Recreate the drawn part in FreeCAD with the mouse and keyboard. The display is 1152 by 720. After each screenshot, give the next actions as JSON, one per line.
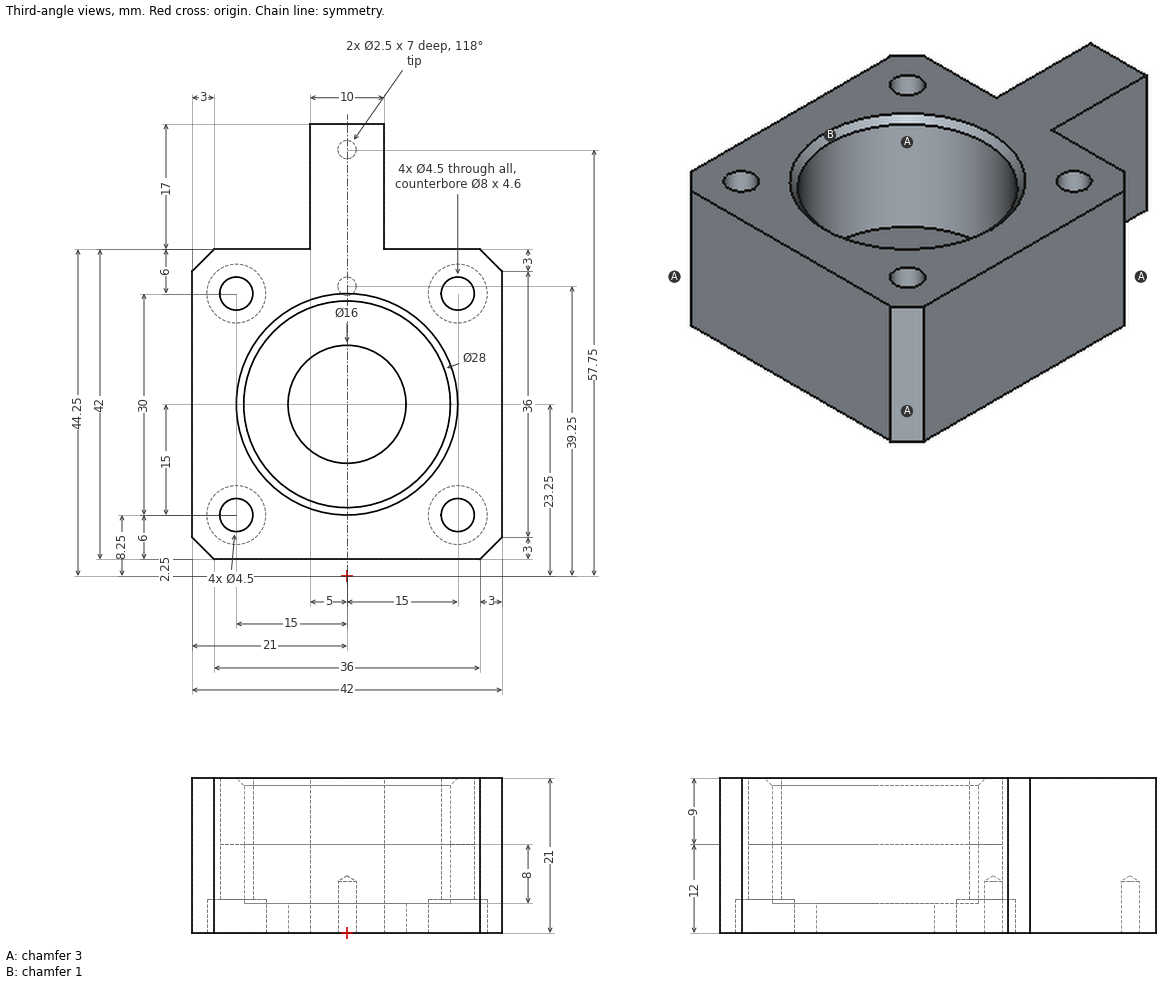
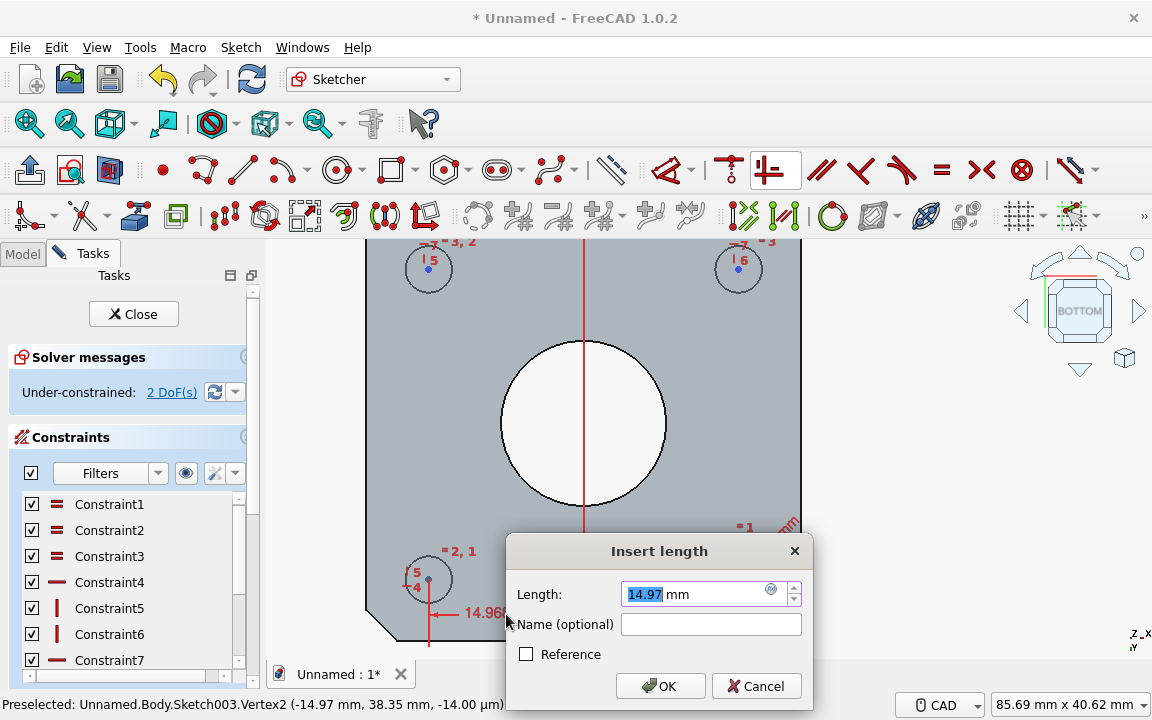
{"action": "type", "text": "15"}
{"action": "key", "text": "Return"}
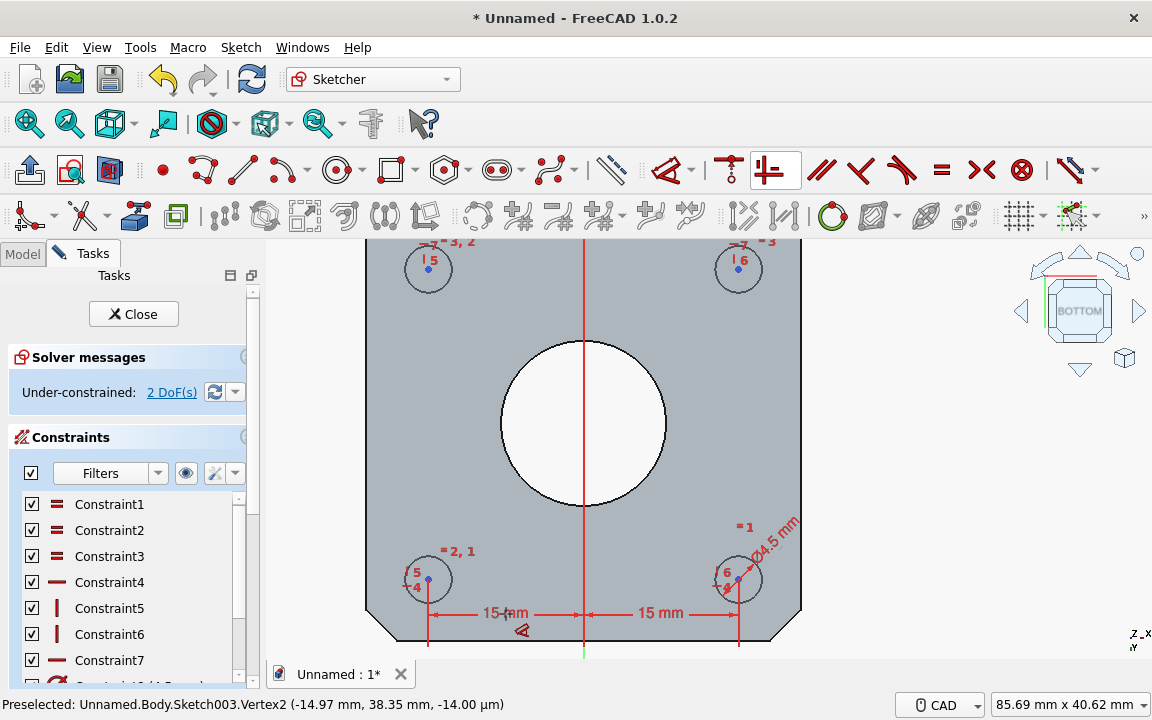
{"action": "left_click", "coordinate": [428, 580]}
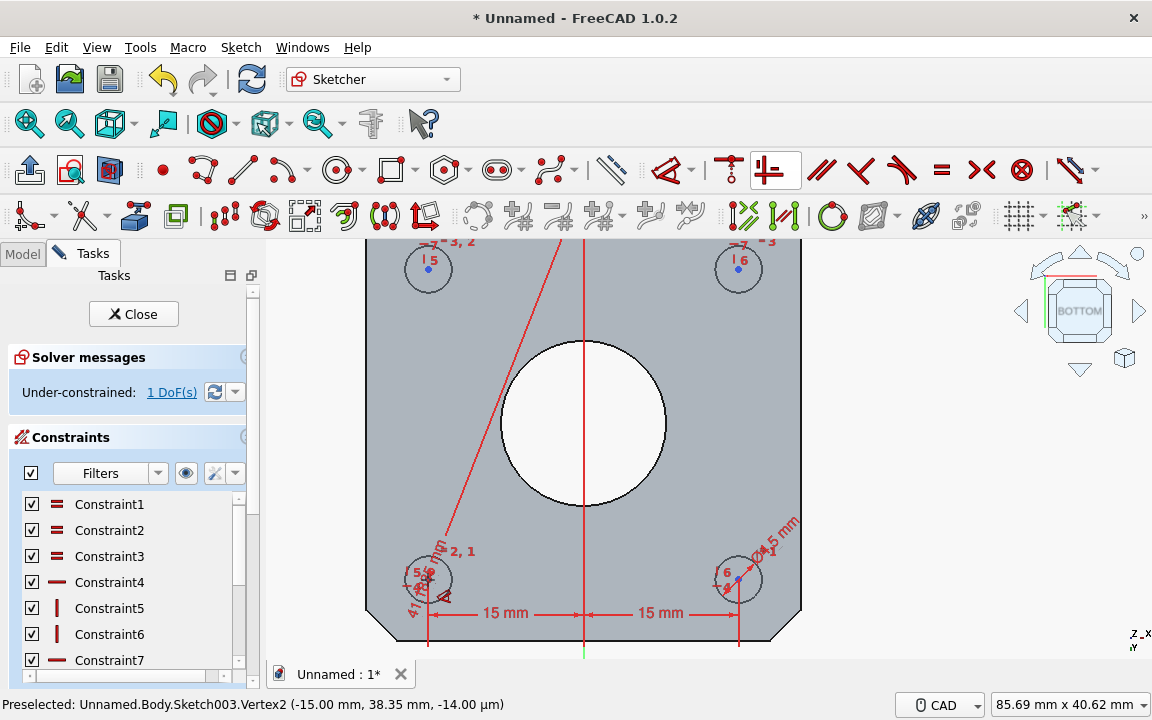
{"action": "left_click", "coordinate": [428, 269]}
{"action": "left_click", "coordinate": [394, 424]}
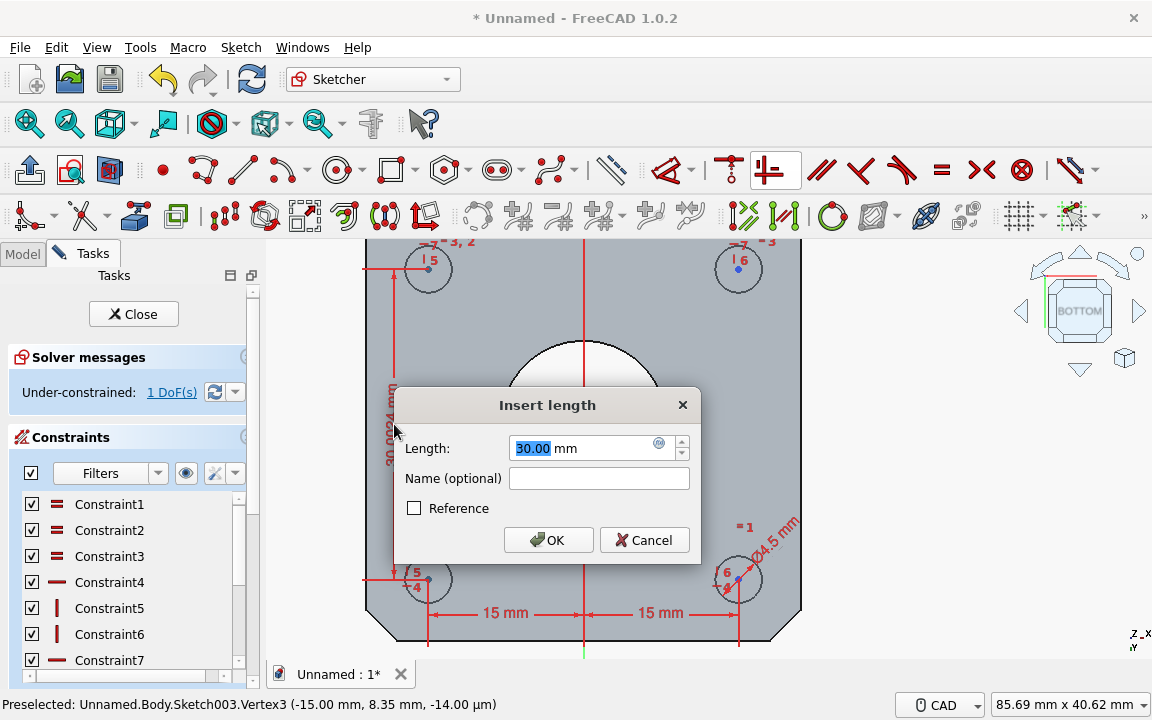
{"action": "type", "text": "30"}
{"action": "key", "text": "Return"}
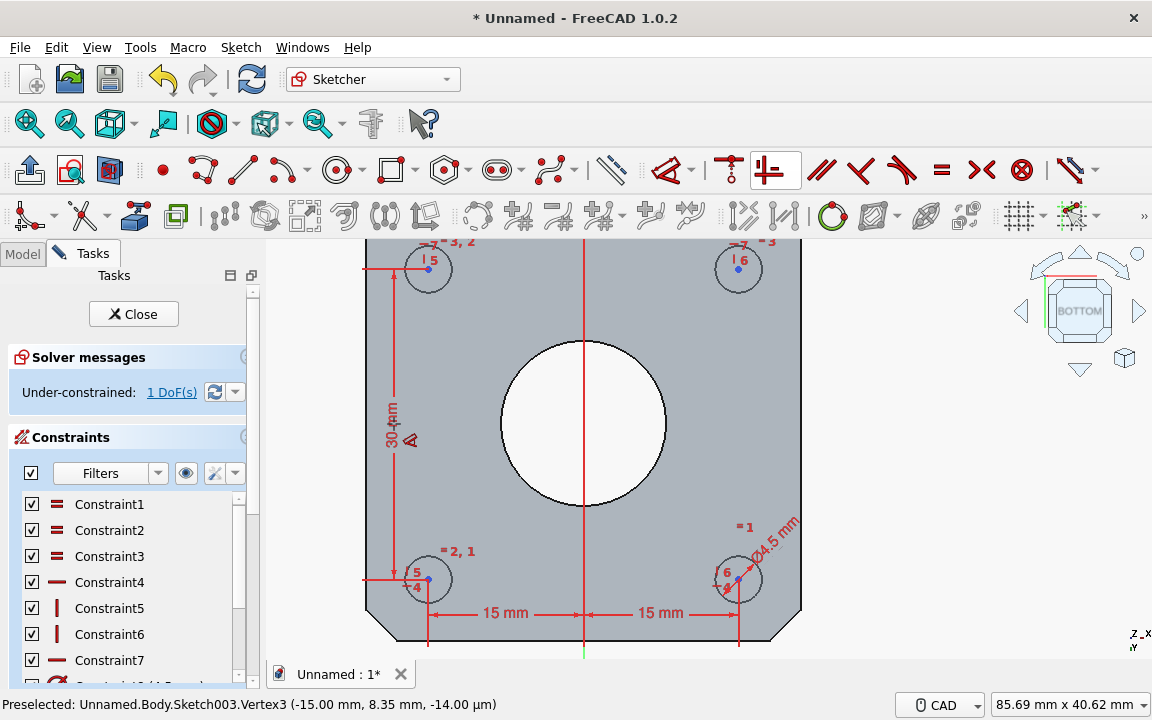
{"action": "left_click", "coordinate": [428, 269]}
{"action": "left_click", "coordinate": [618, 268]}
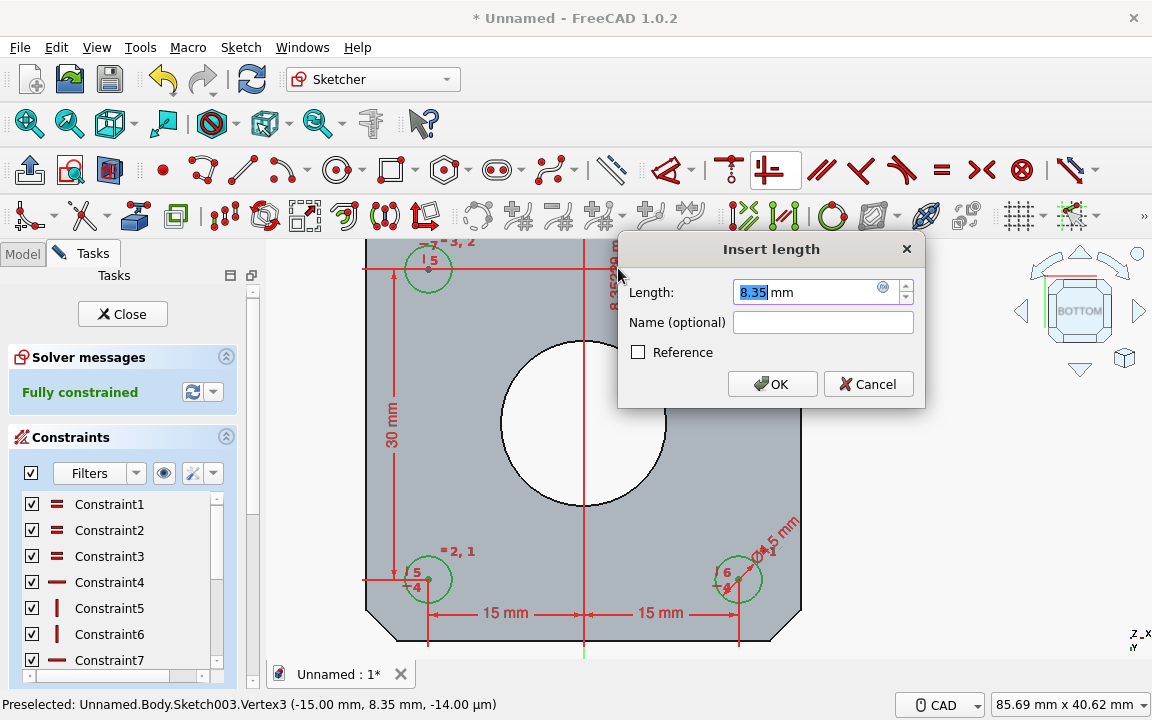
{"action": "type", "text": "8.25"}
{"action": "key", "text": "Return"}
{"action": "key", "text": "Escape"}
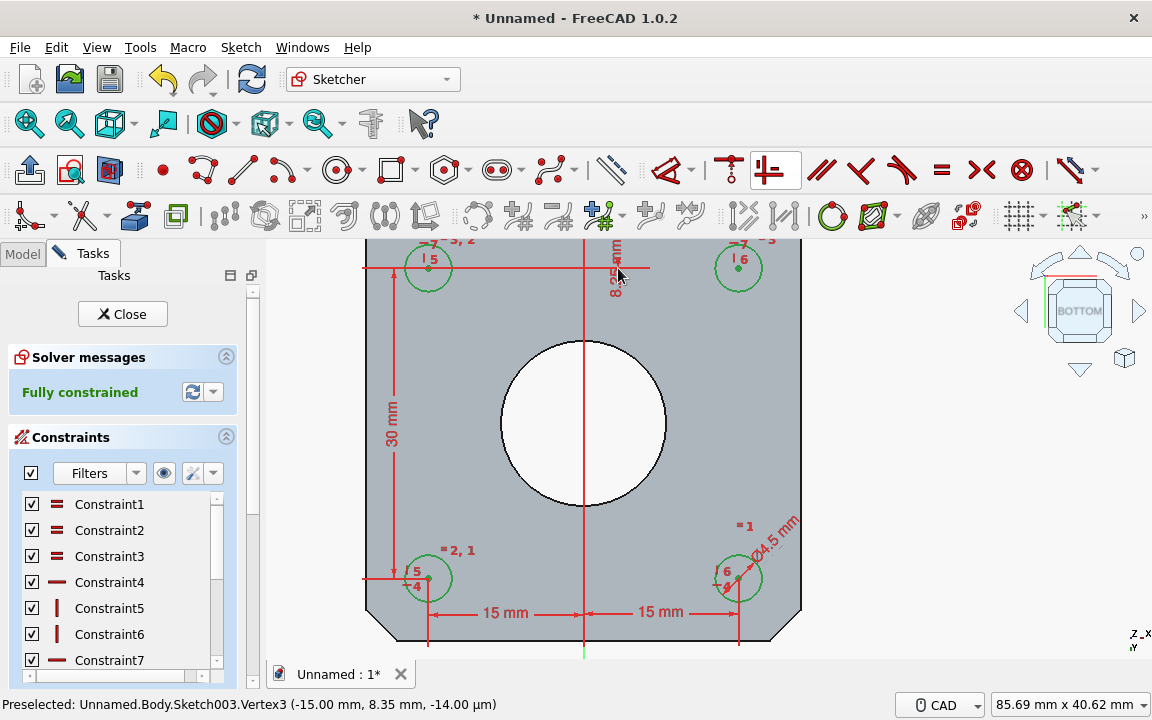
{"action": "left_click", "coordinate": [123, 314]}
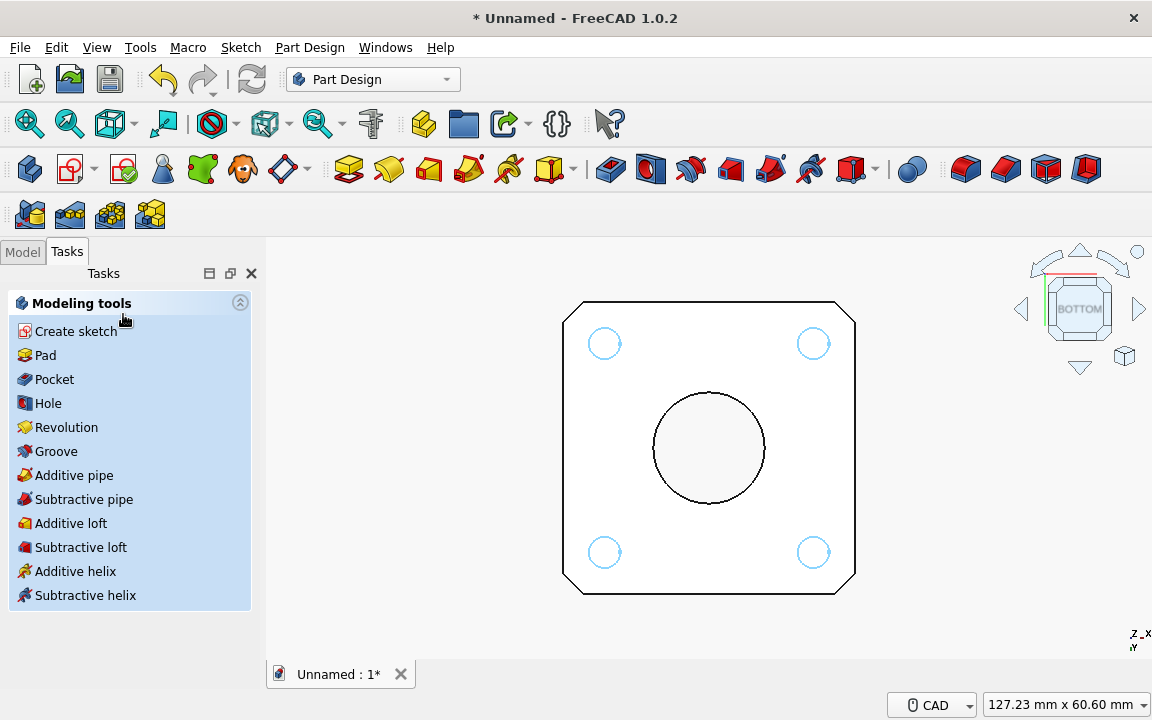
{"action": "left_click", "coordinate": [652, 170]}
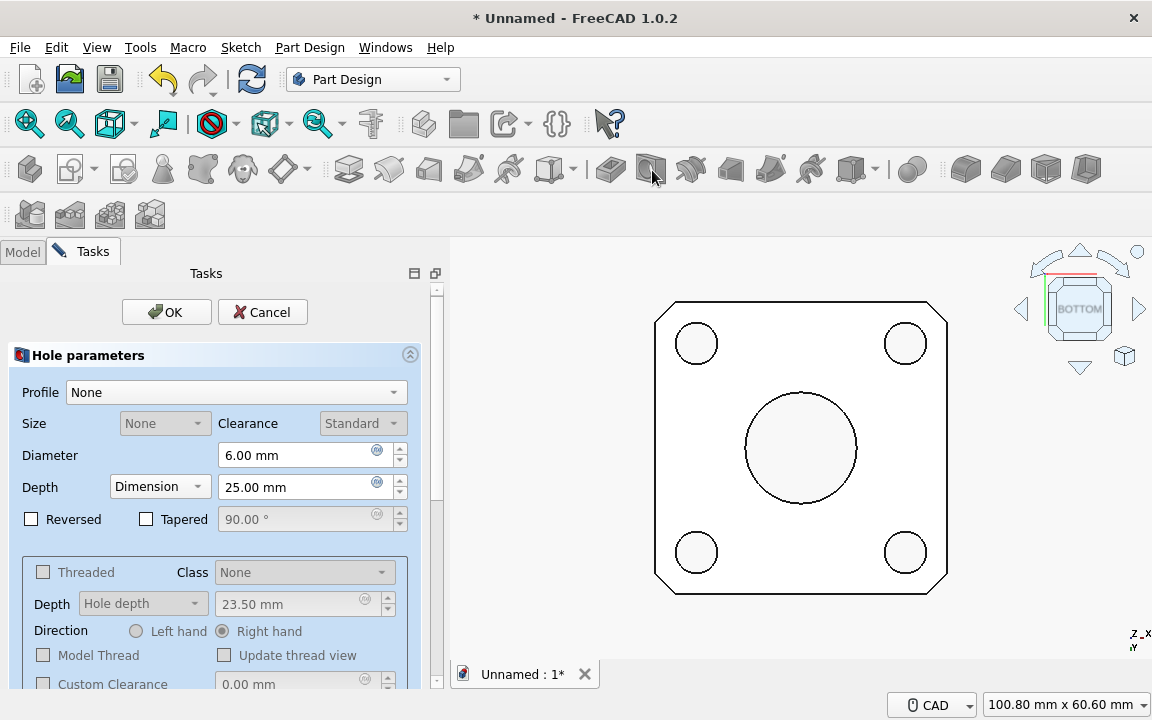
{"action": "triple_click", "coordinate": [305, 455]}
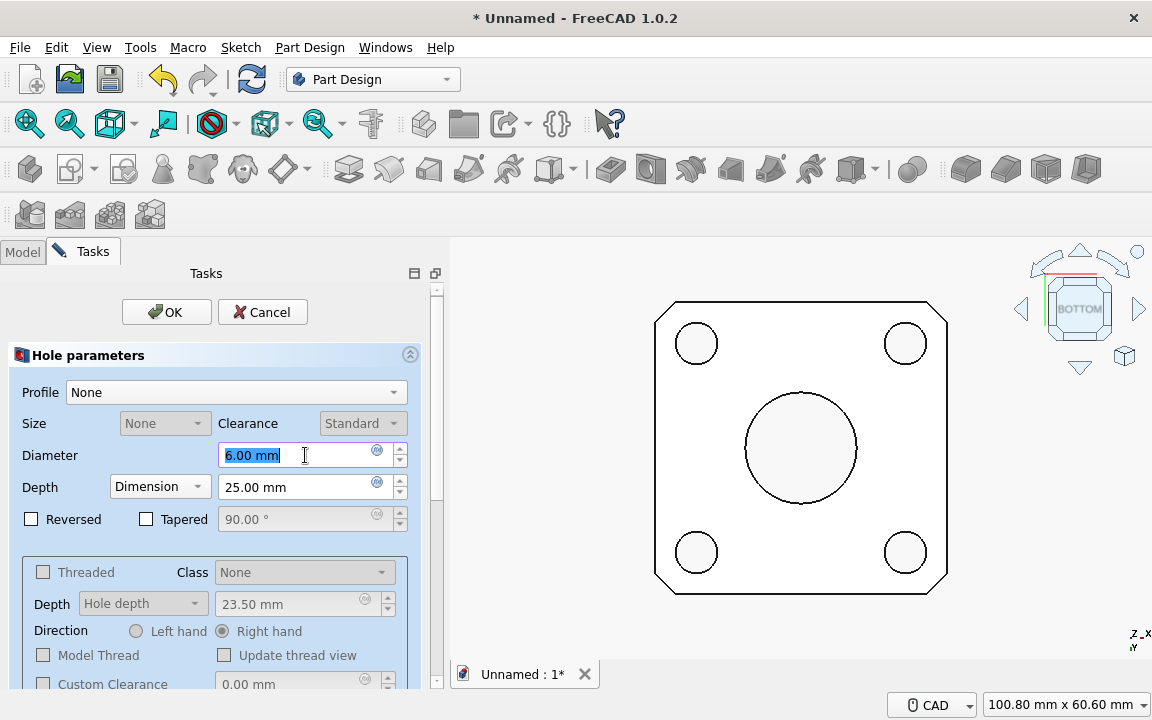
{"action": "type", "text": "4.5"}
{"action": "key", "text": "Tab"}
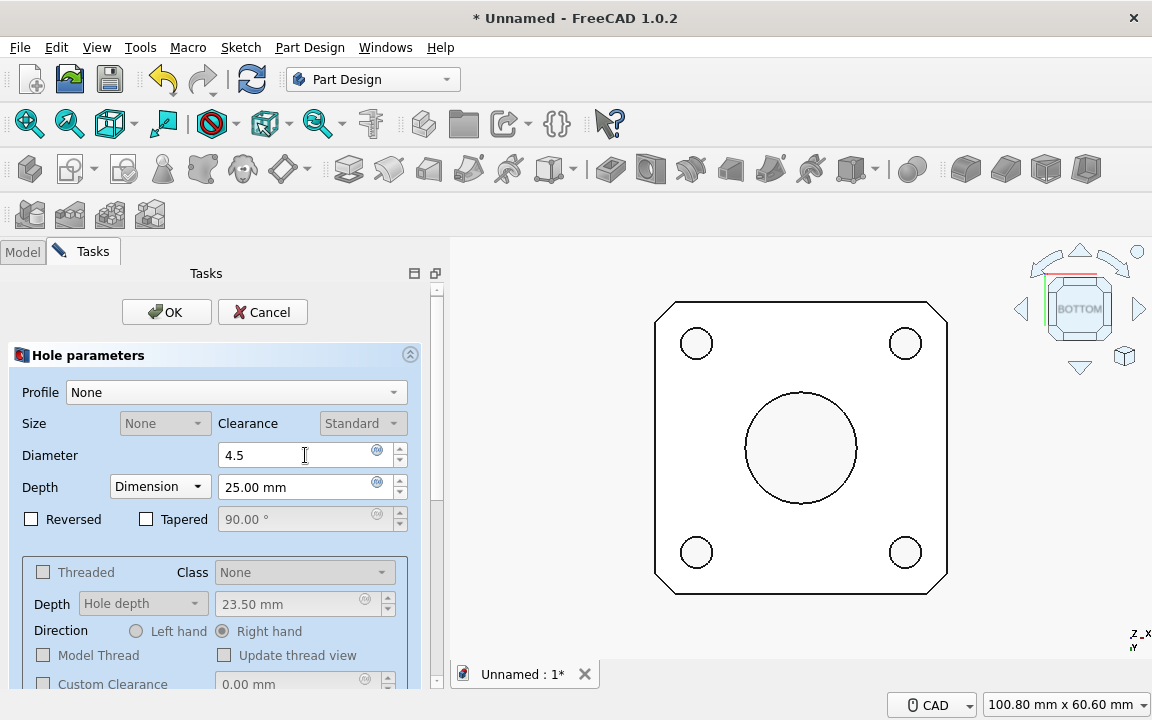
{"action": "left_click", "coordinate": [161, 486]}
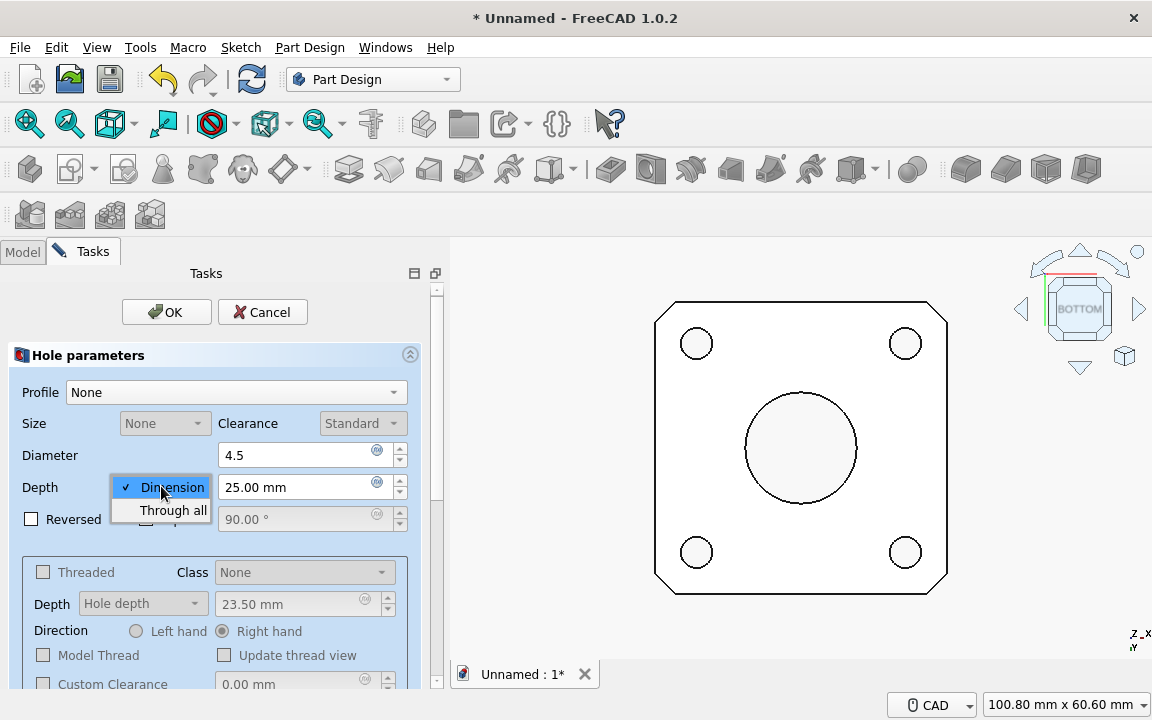
{"action": "left_click", "coordinate": [160, 510]}